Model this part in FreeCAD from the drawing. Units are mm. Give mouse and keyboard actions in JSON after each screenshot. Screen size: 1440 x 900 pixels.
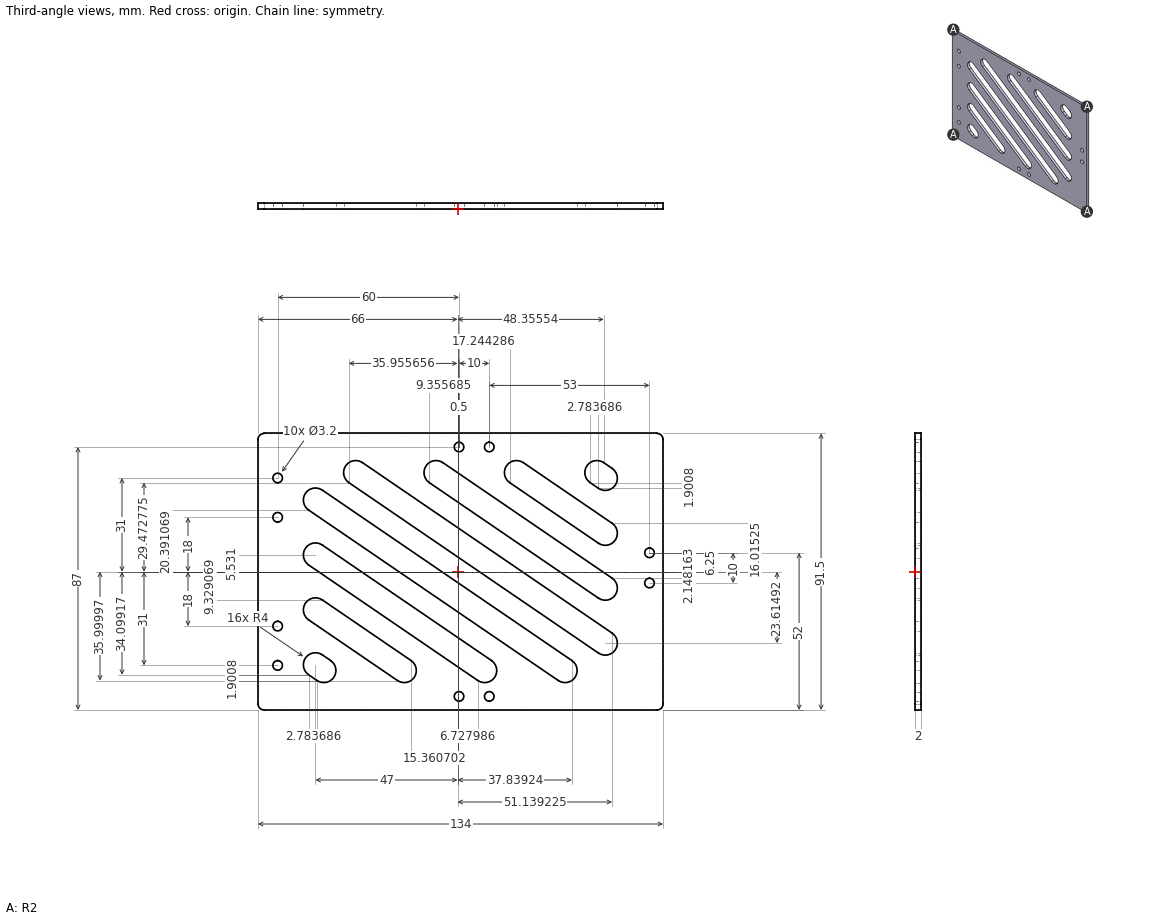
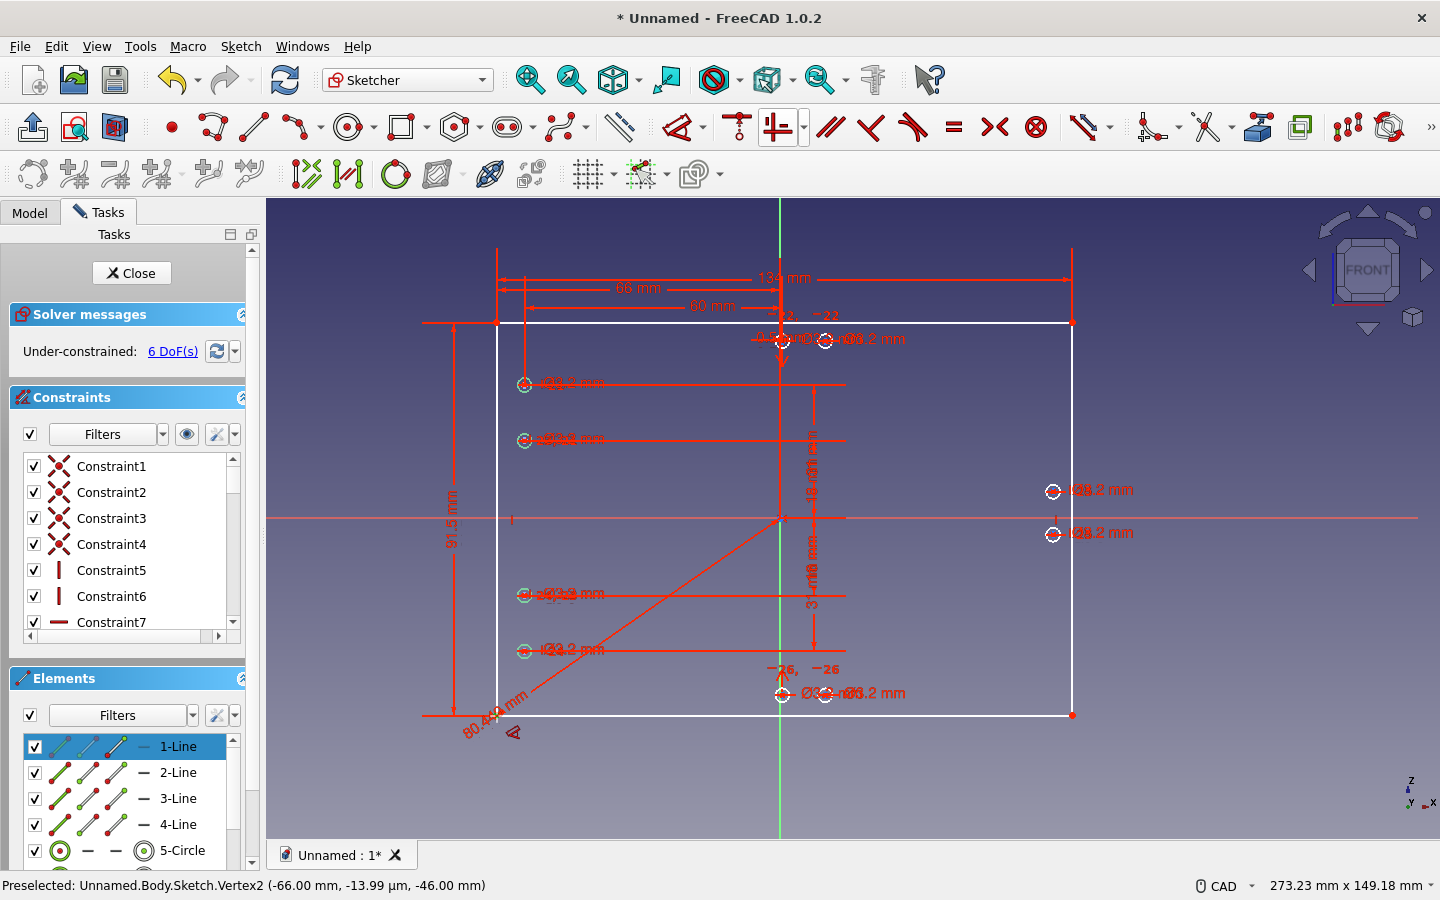
{"action": "left_click", "coordinate": [782, 341]}
{"action": "left_click", "coordinate": [463, 442]}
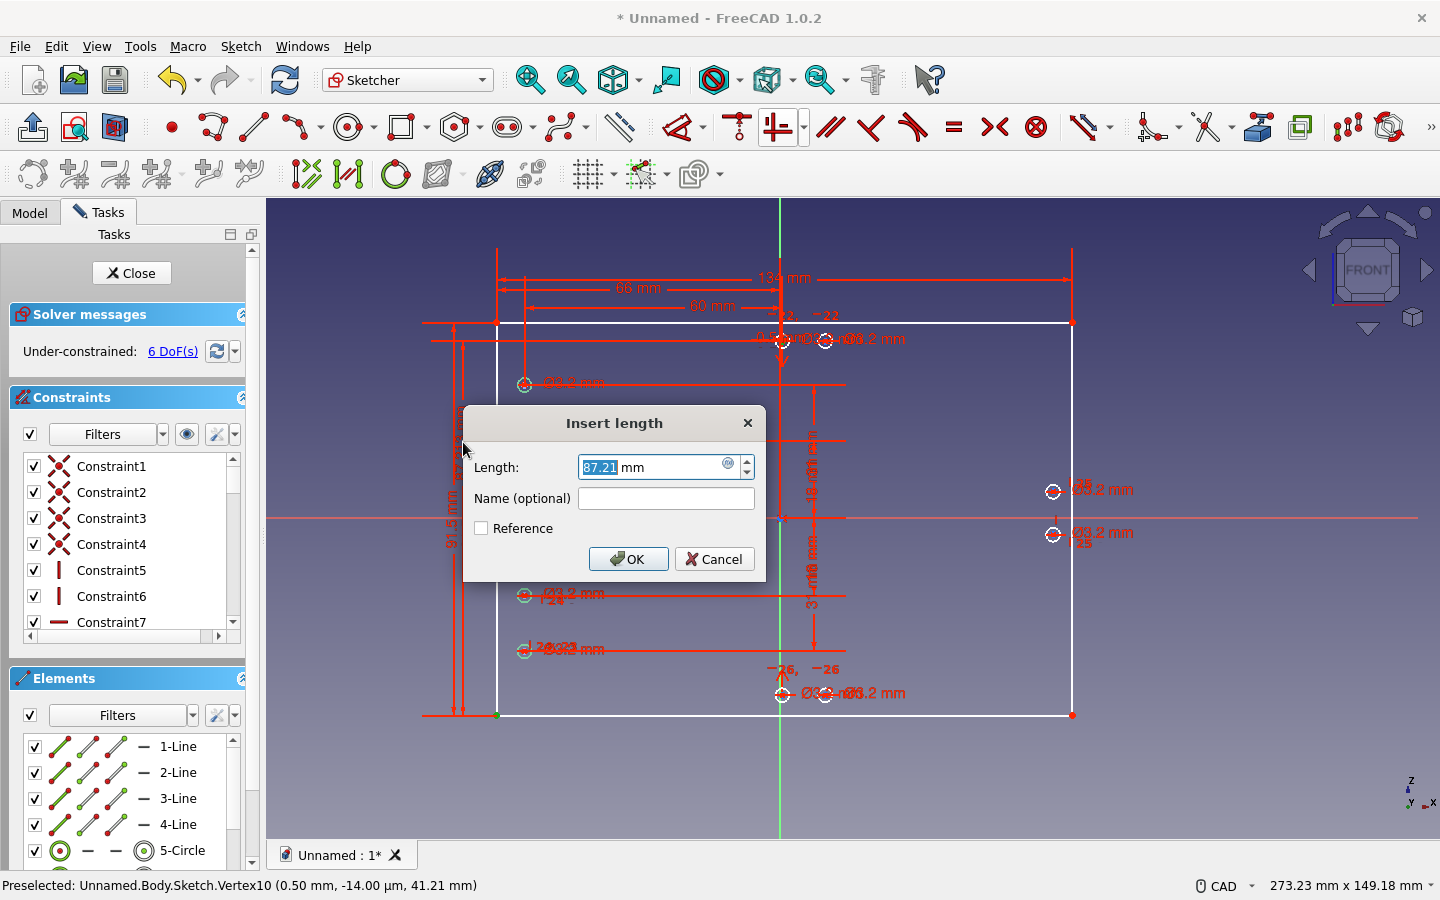
{"action": "type", "text": "87"}
{"action": "key", "text": "Return"}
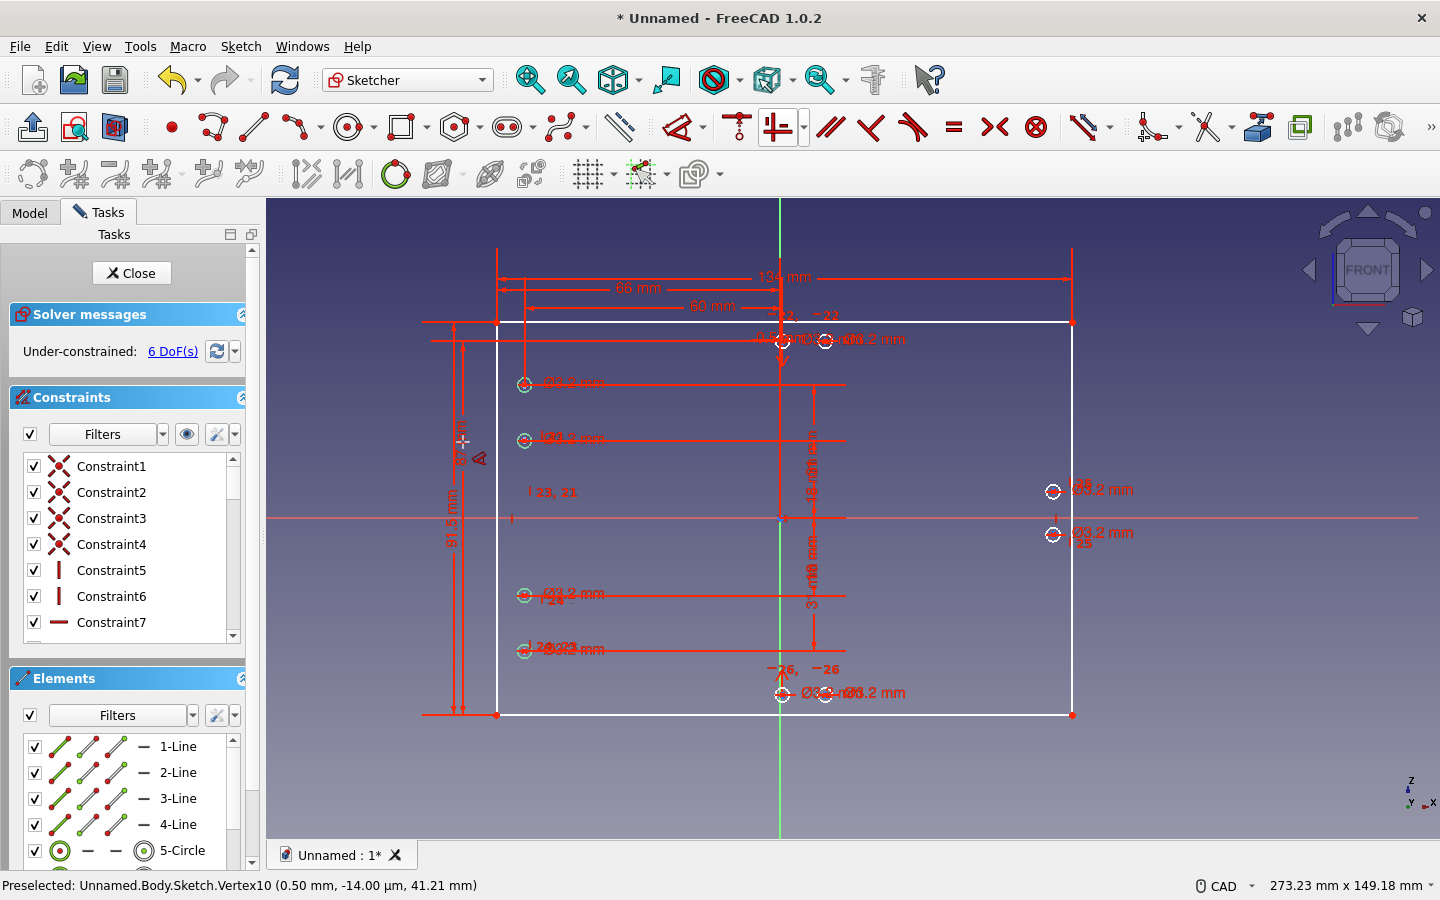
{"action": "left_click", "coordinate": [782, 341]}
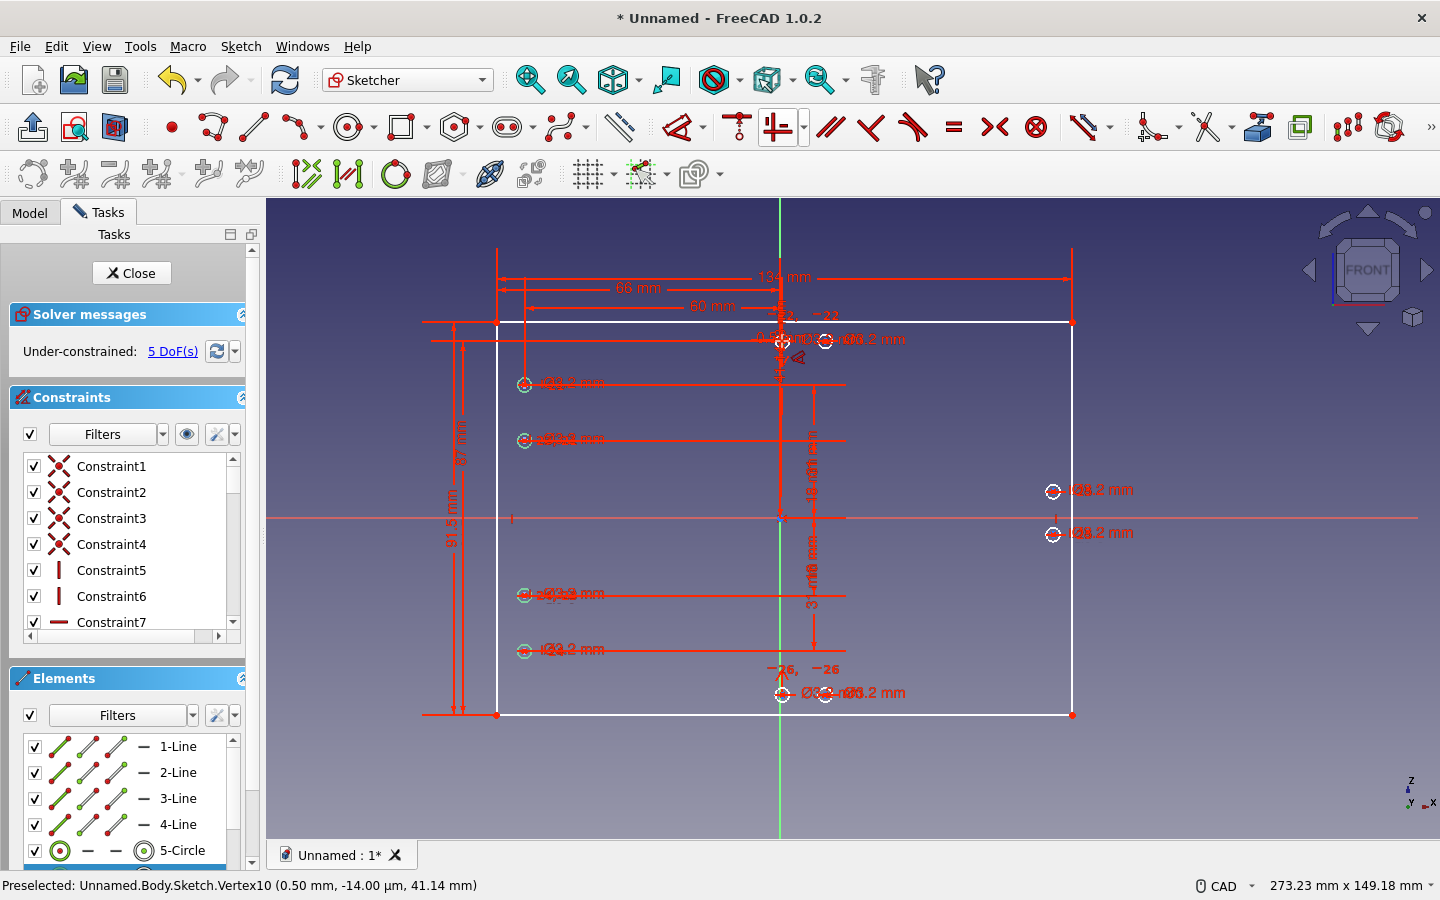
{"action": "left_click", "coordinate": [825, 341]}
{"action": "left_click", "coordinate": [804, 307]}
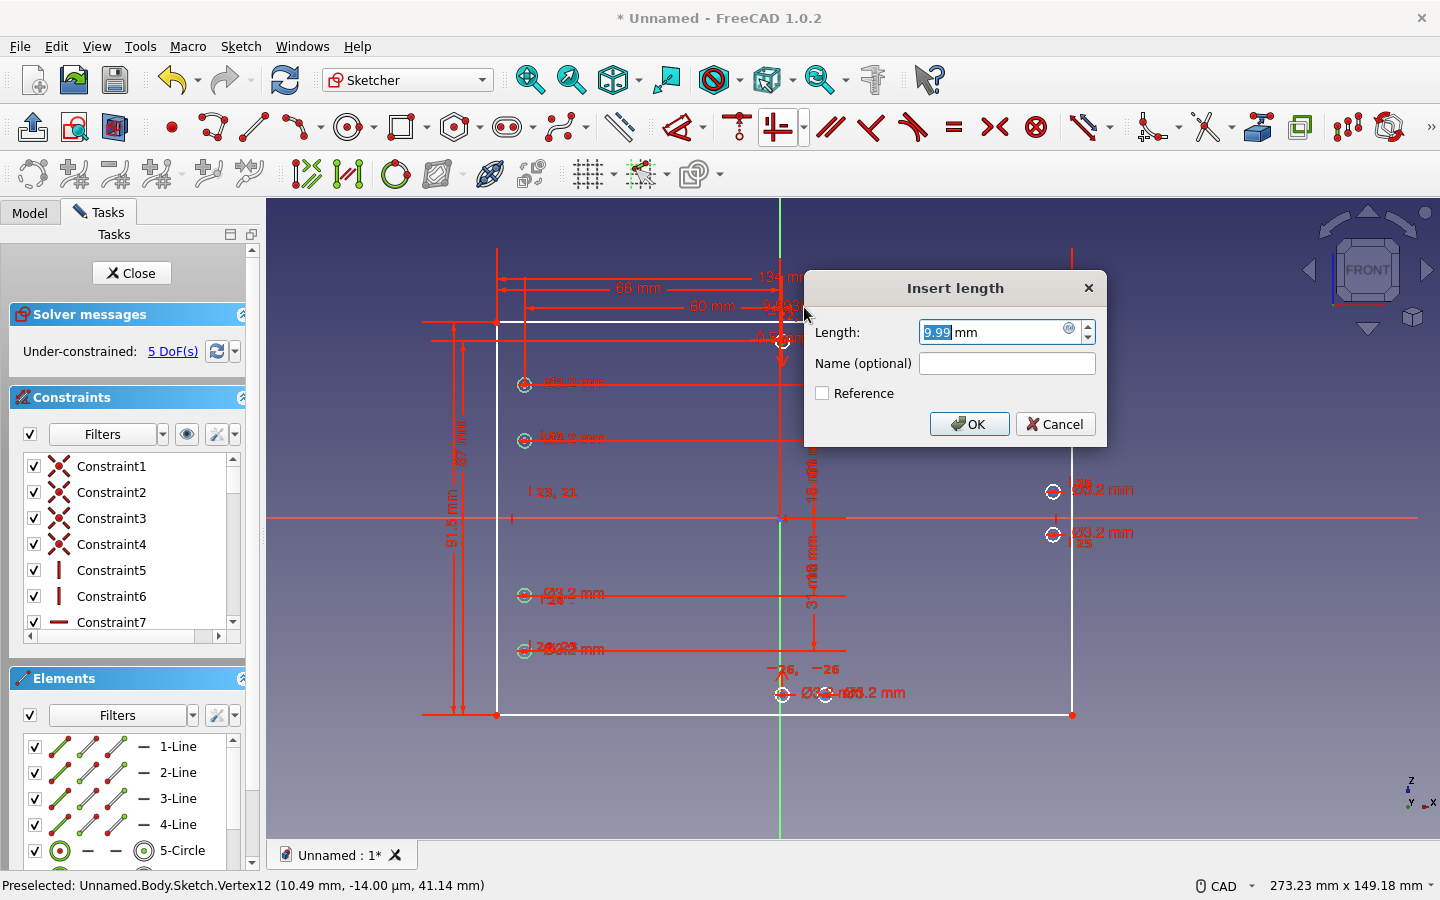
{"action": "type", "text": "10"}
{"action": "key", "text": "Return"}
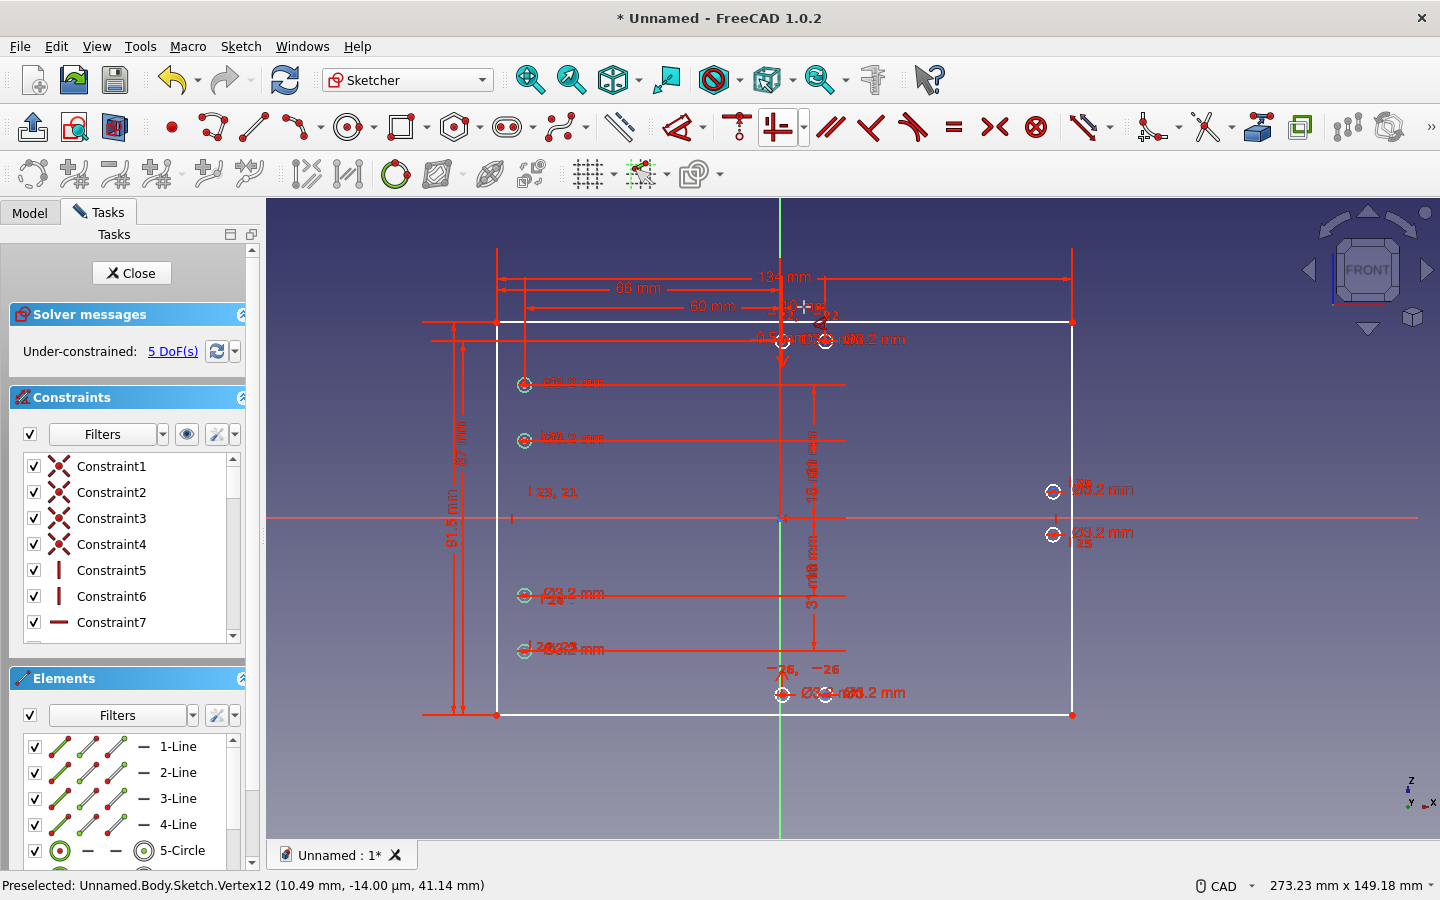
{"action": "left_click", "coordinate": [825, 341]}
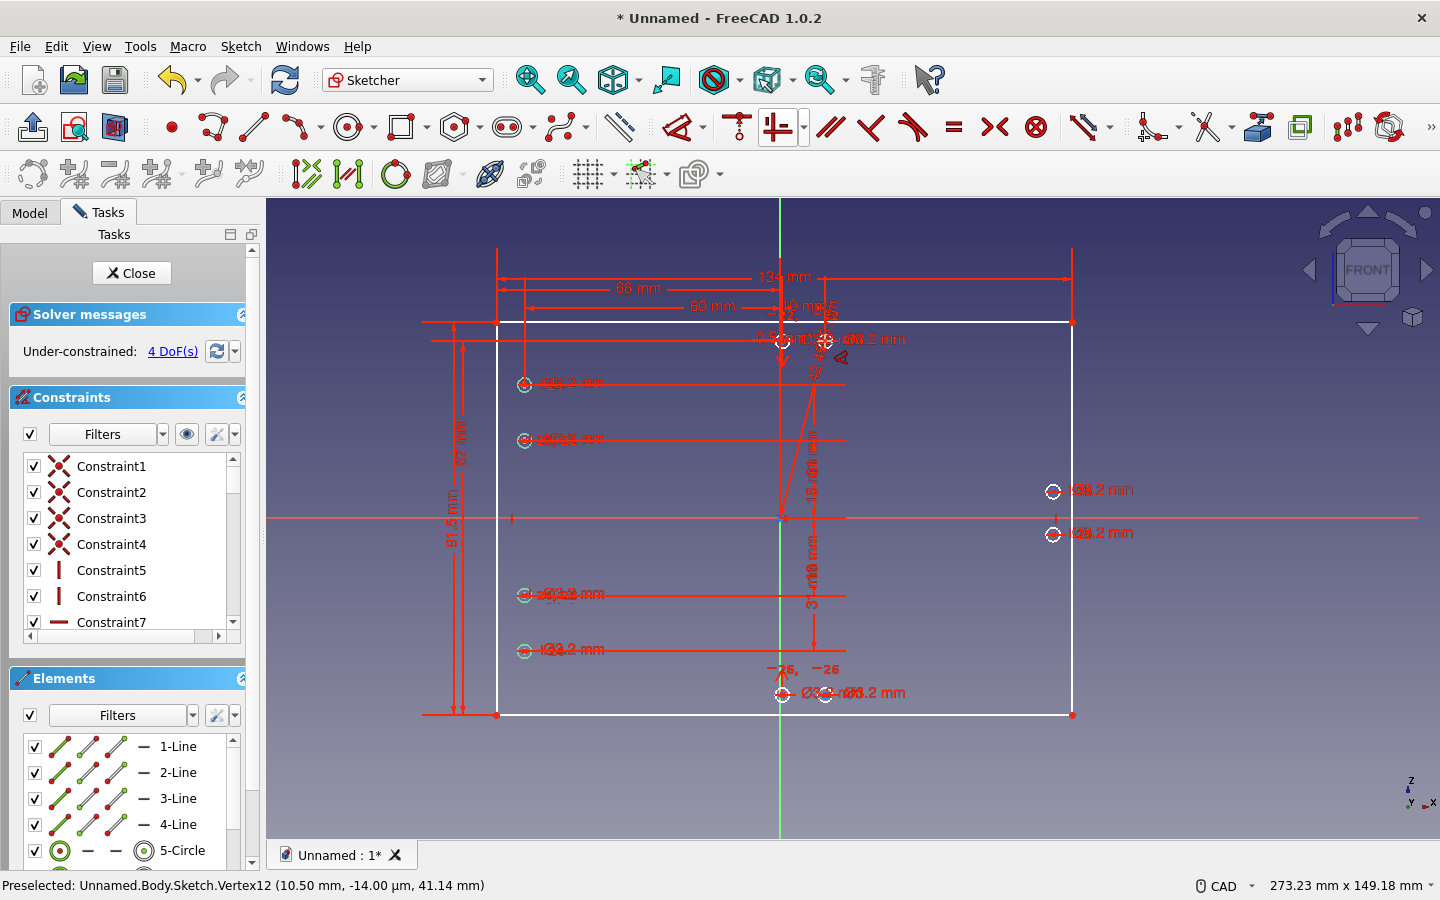
{"action": "left_click", "coordinate": [1053, 492]}
{"action": "left_click", "coordinate": [939, 307]}